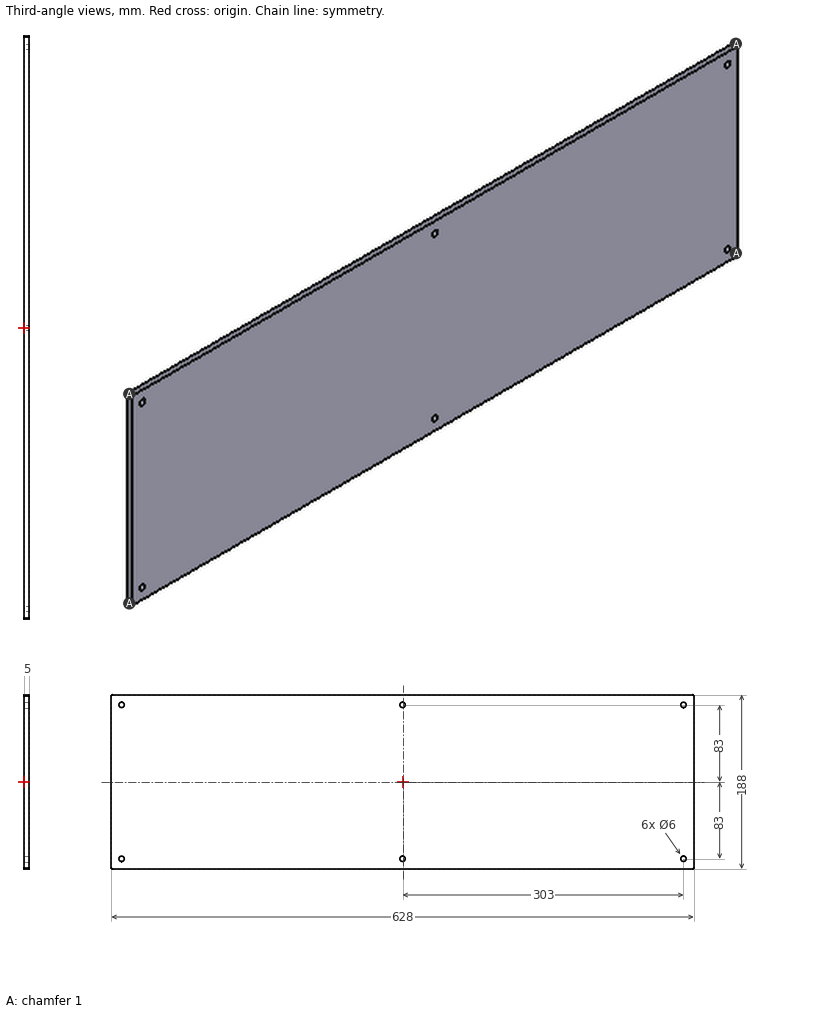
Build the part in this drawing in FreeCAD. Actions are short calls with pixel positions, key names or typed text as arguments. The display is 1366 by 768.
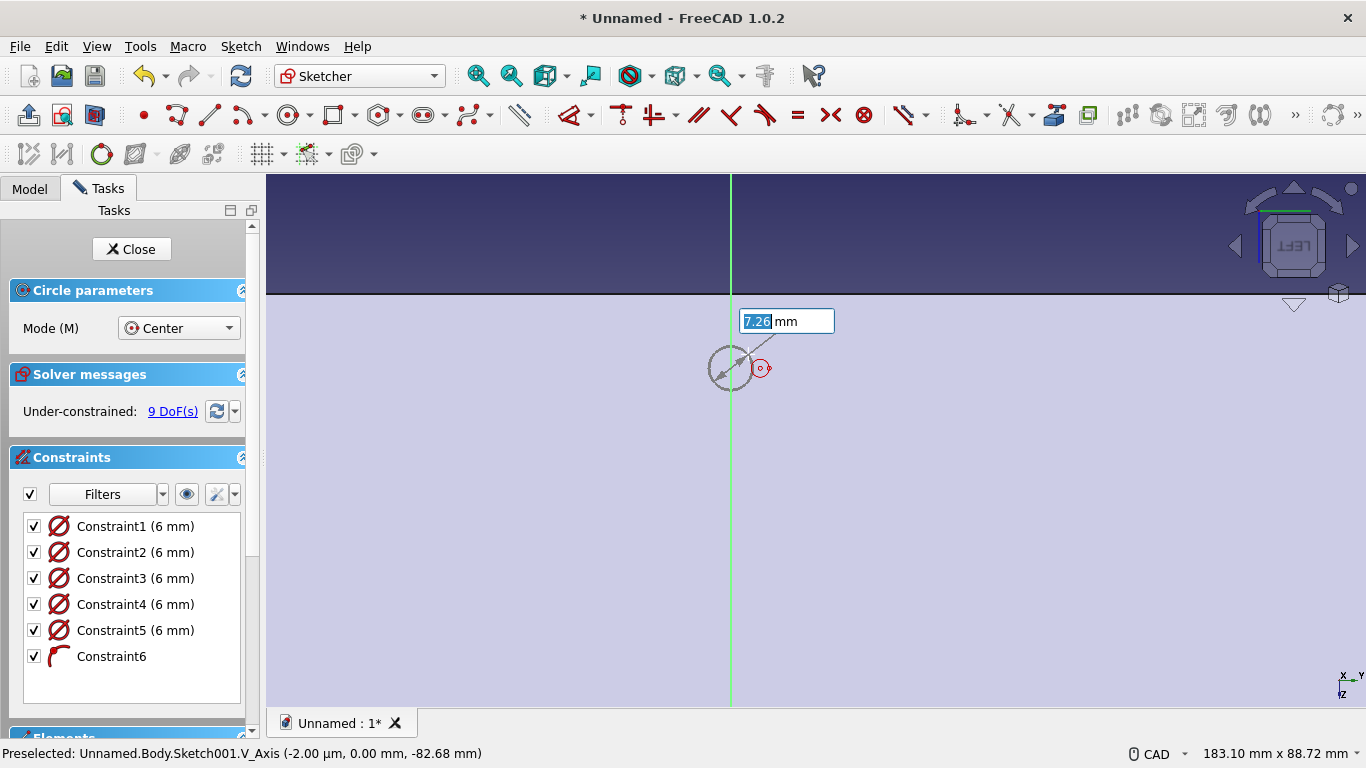
text(6)
key(Return)
key(Escape)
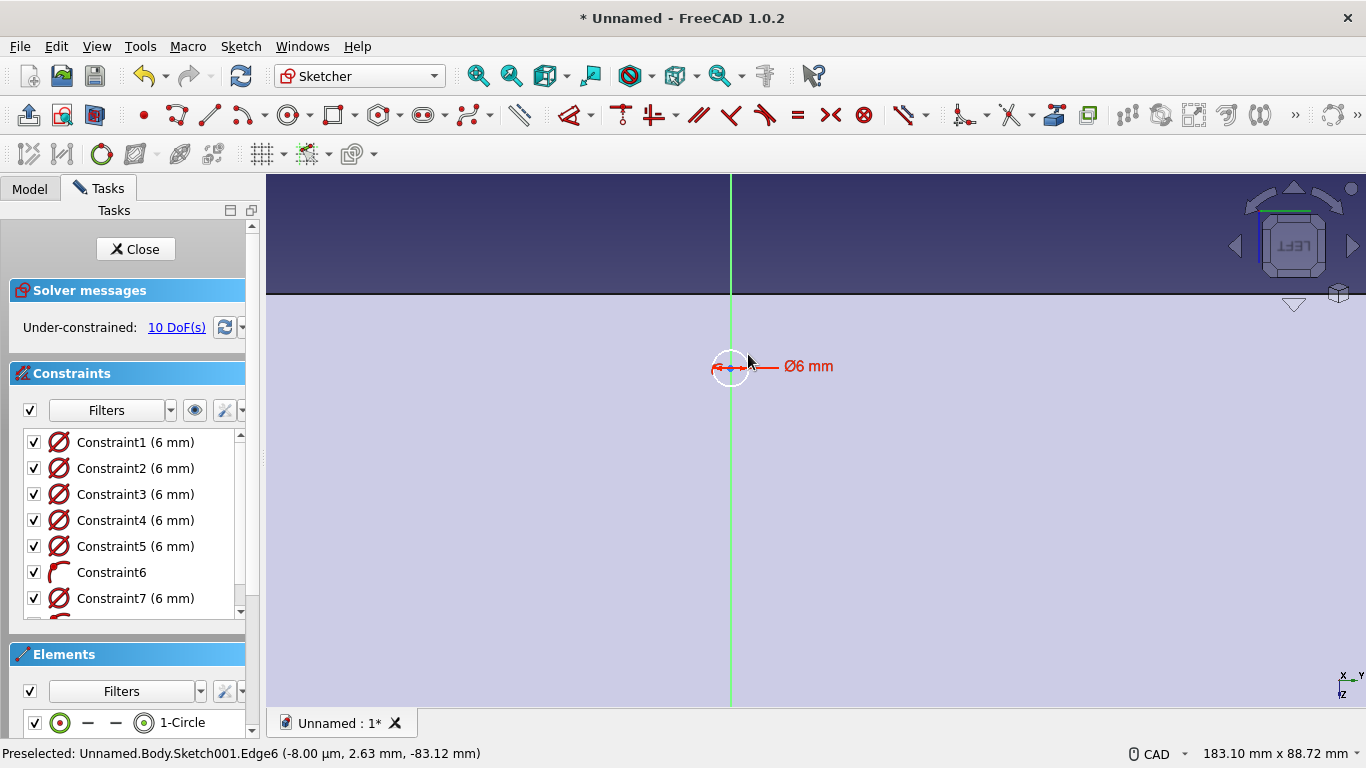
scroll(751, 358, down, 9)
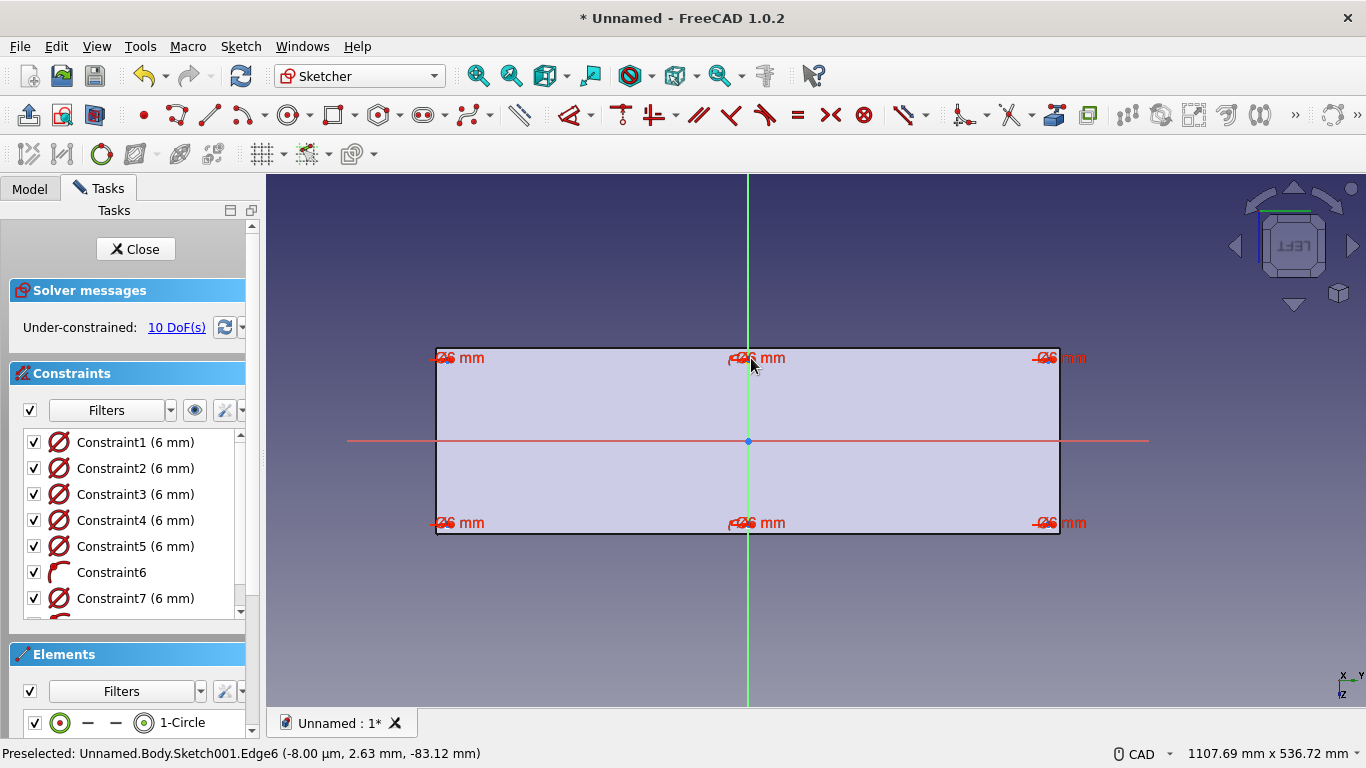
click(1049, 360)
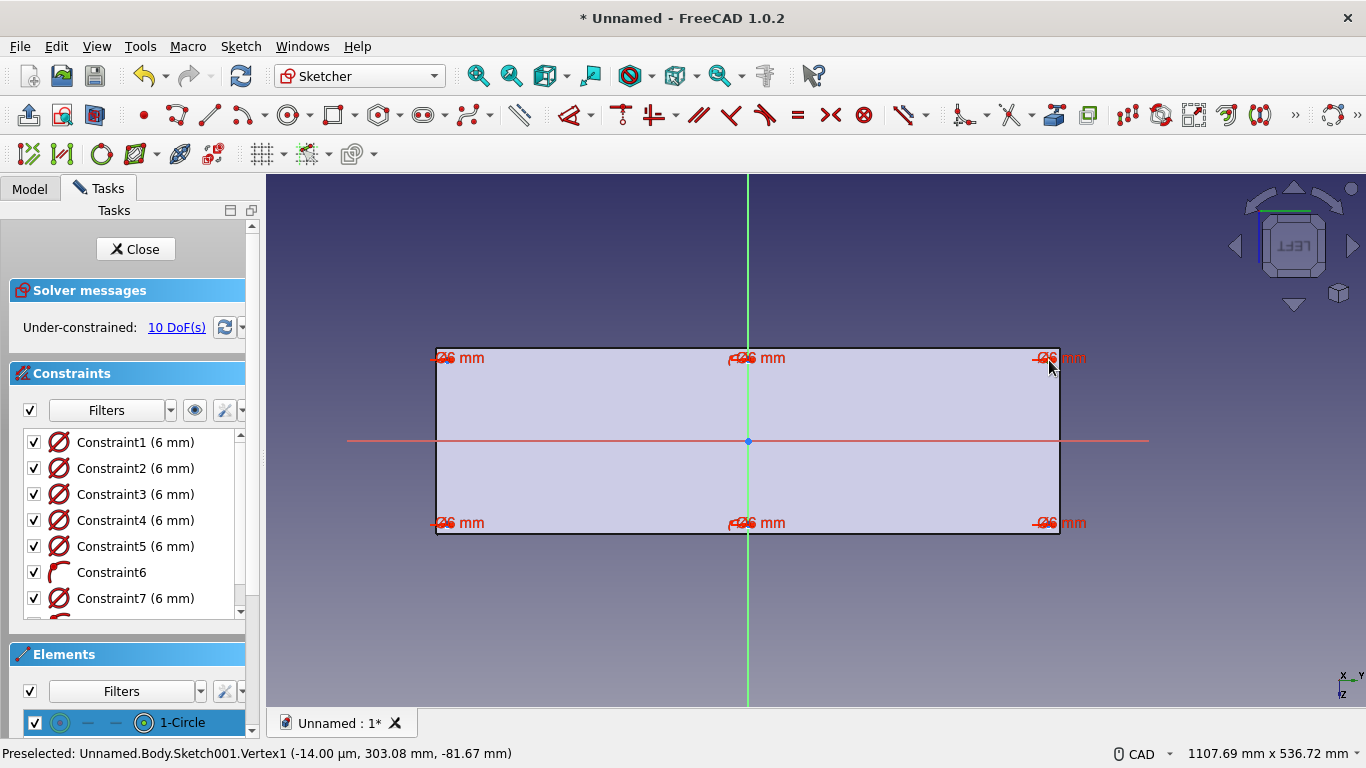
click(447, 360)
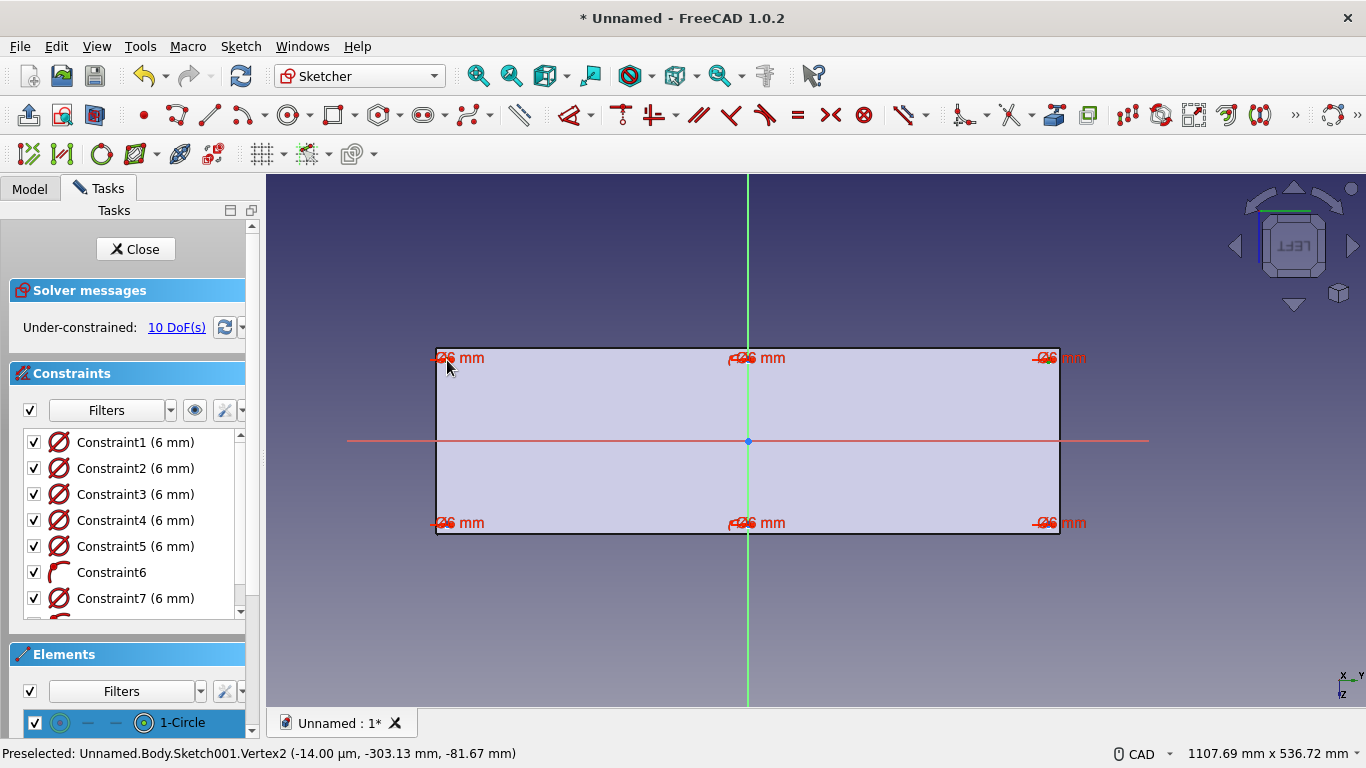
click(748, 645)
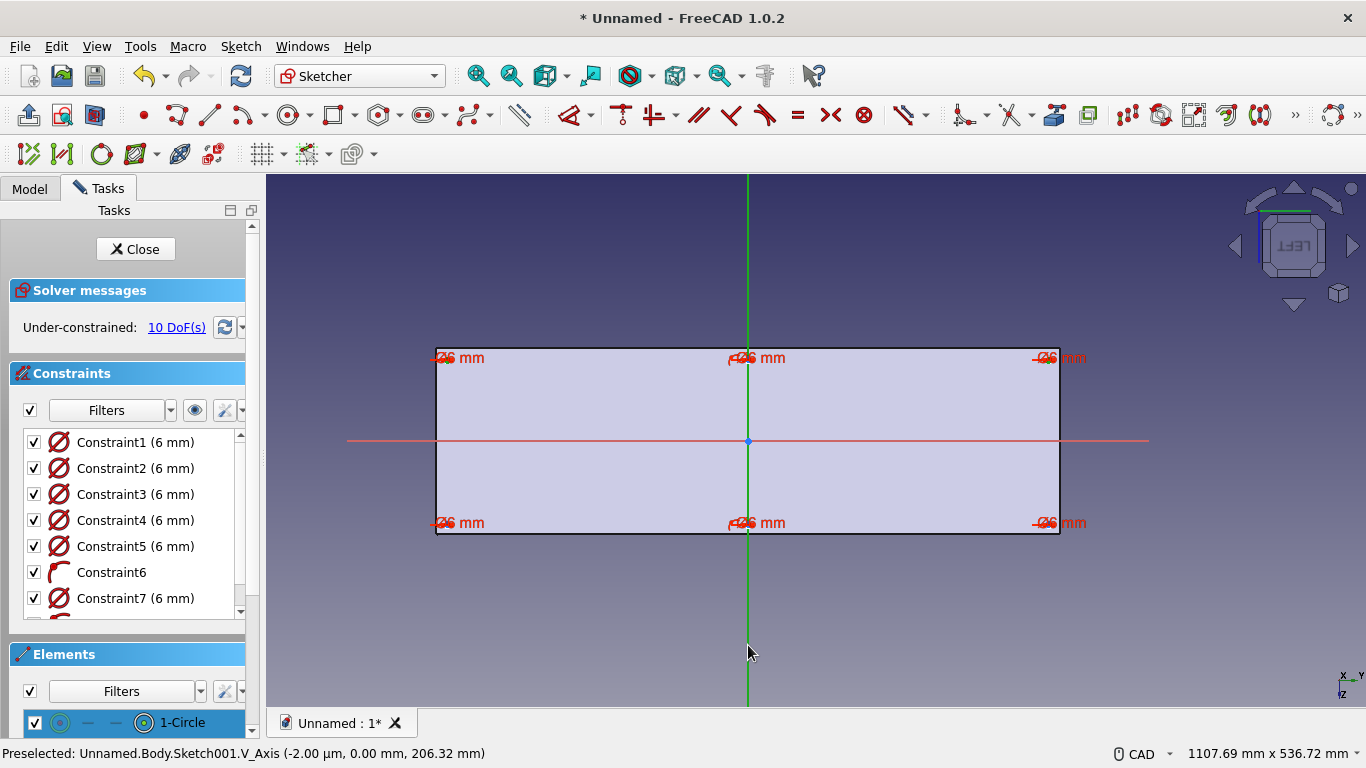
key(s)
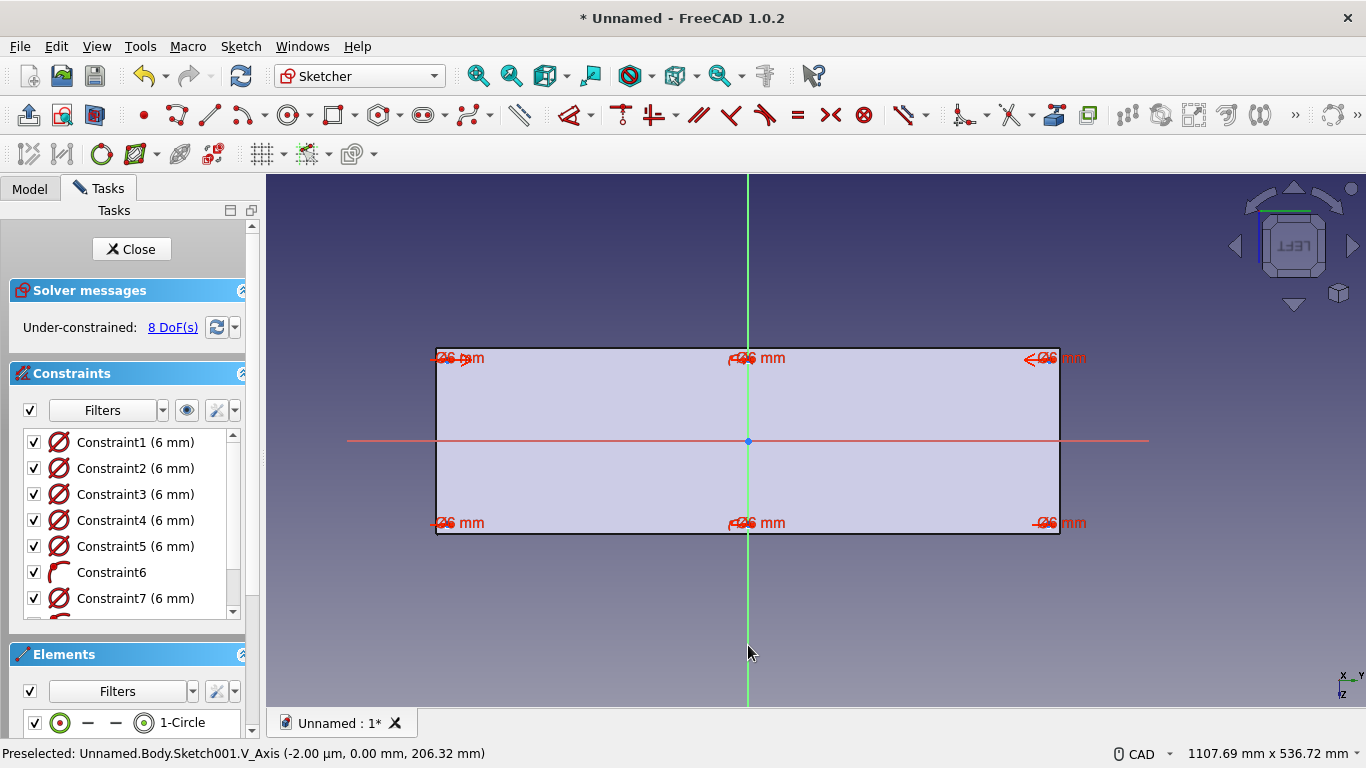
click(447, 360)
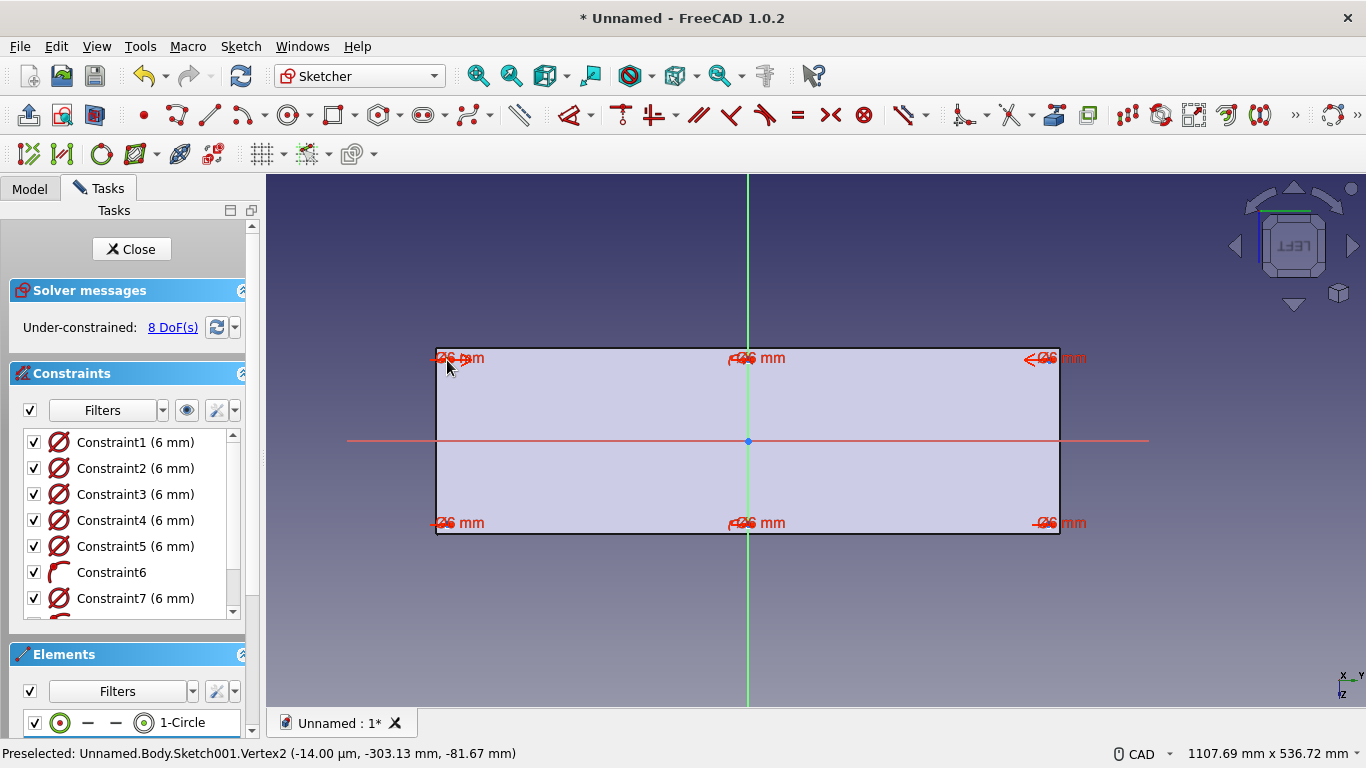
click(447, 525)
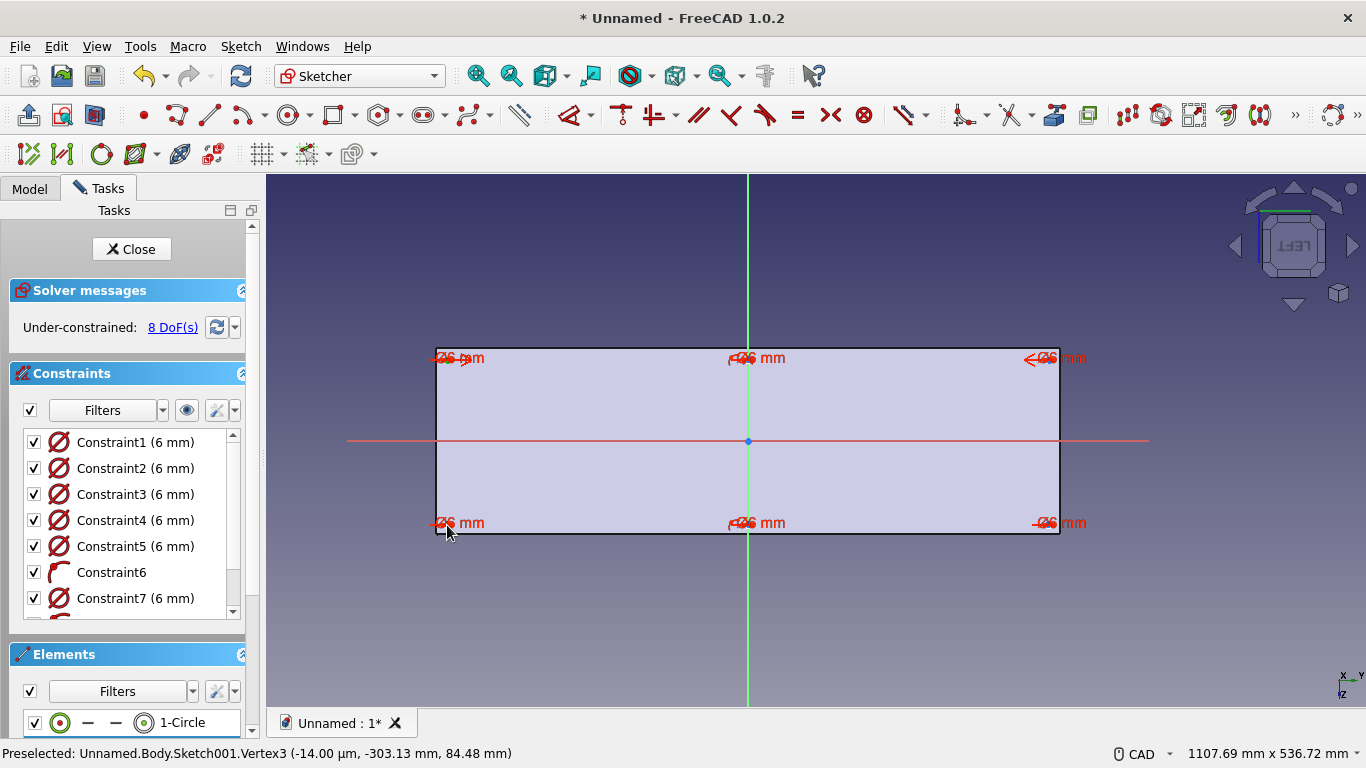
click(359, 441)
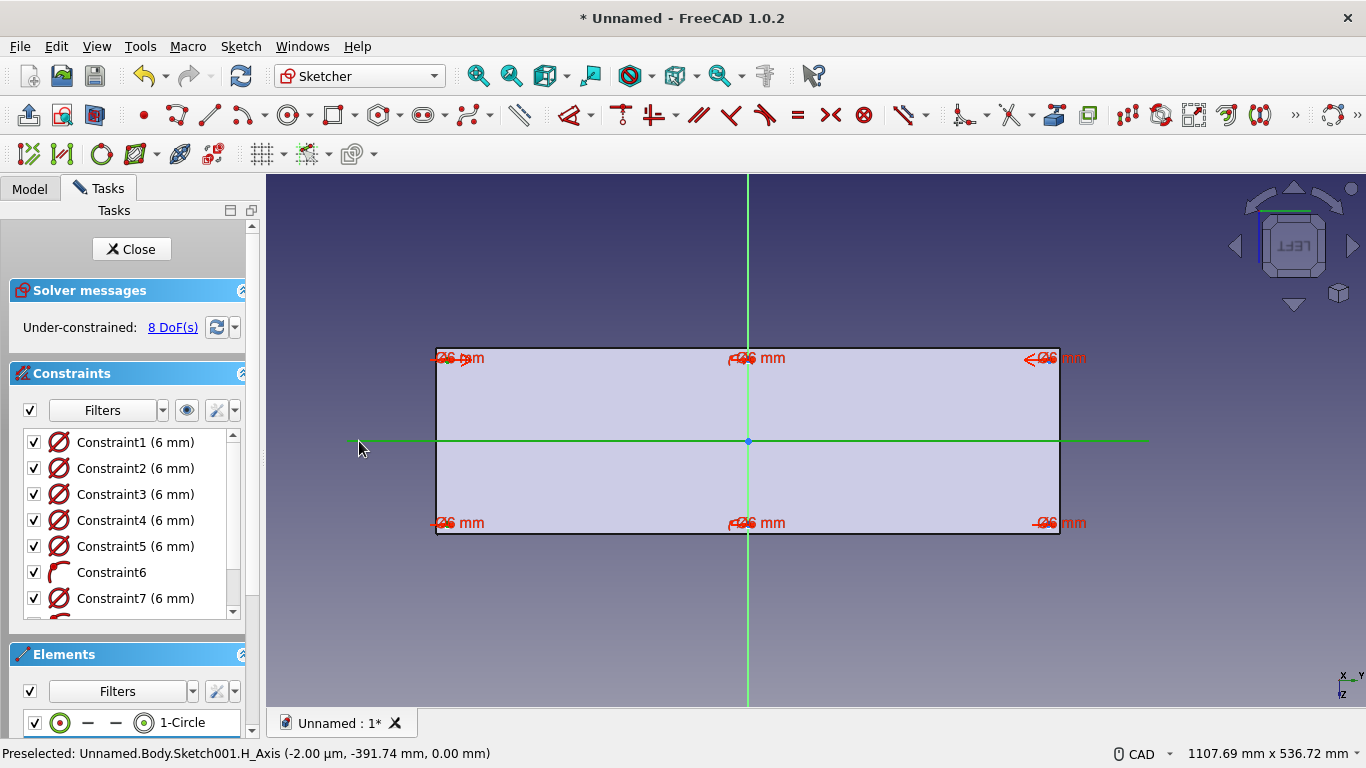
click(831, 116)